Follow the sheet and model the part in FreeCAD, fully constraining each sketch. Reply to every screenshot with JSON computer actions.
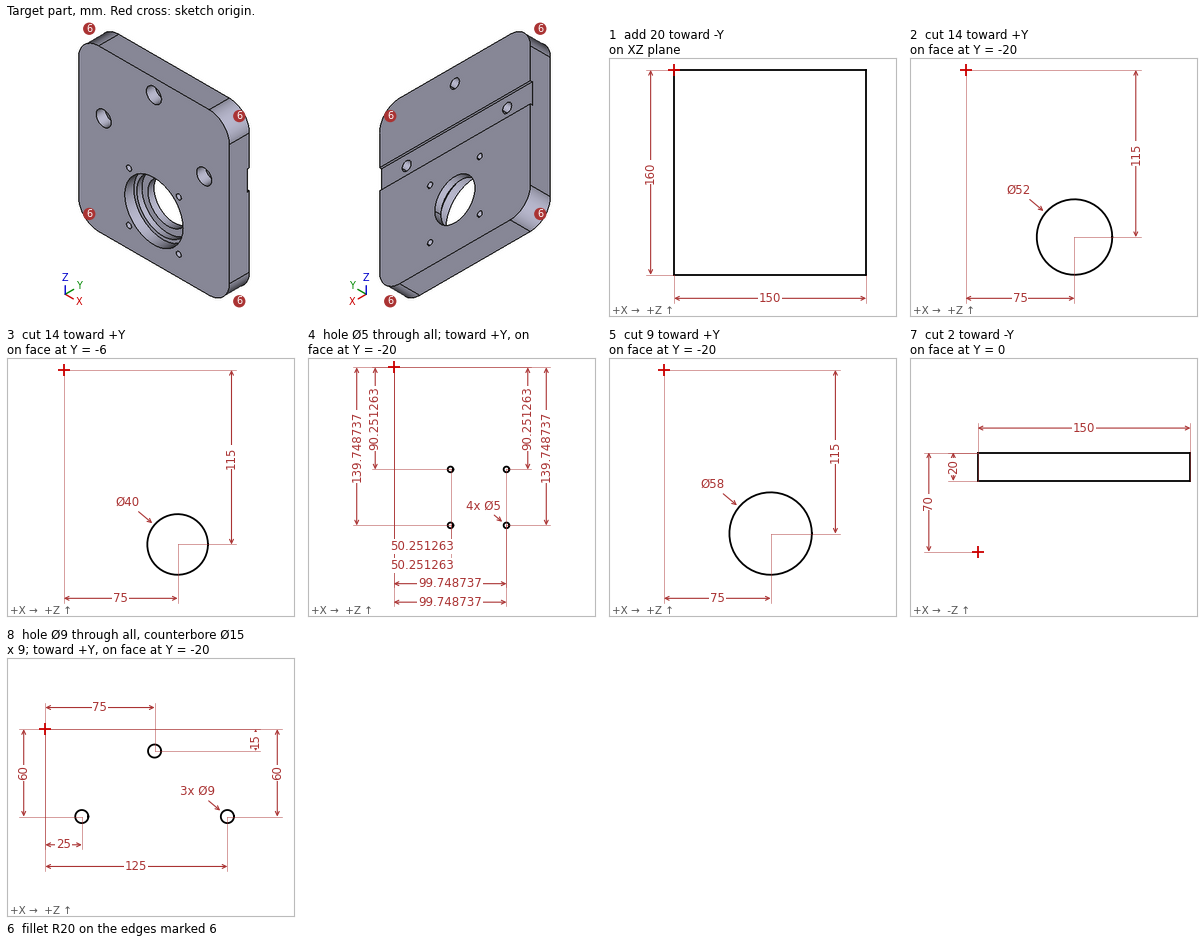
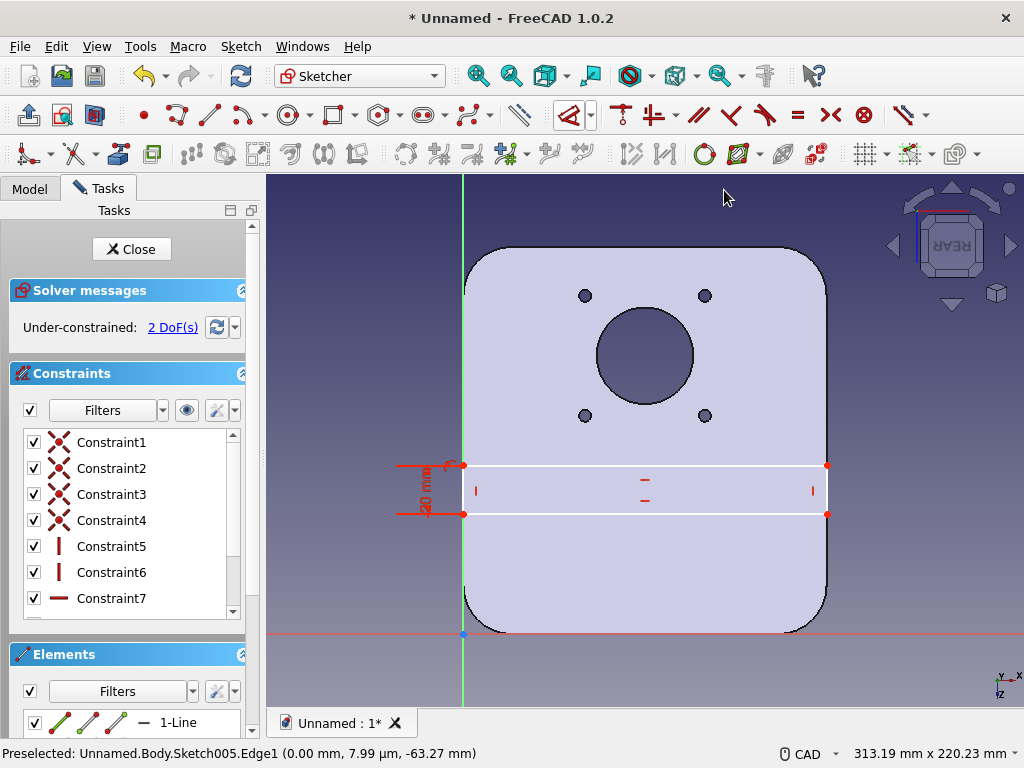
{"action": "left_click", "coordinate": [573, 514]}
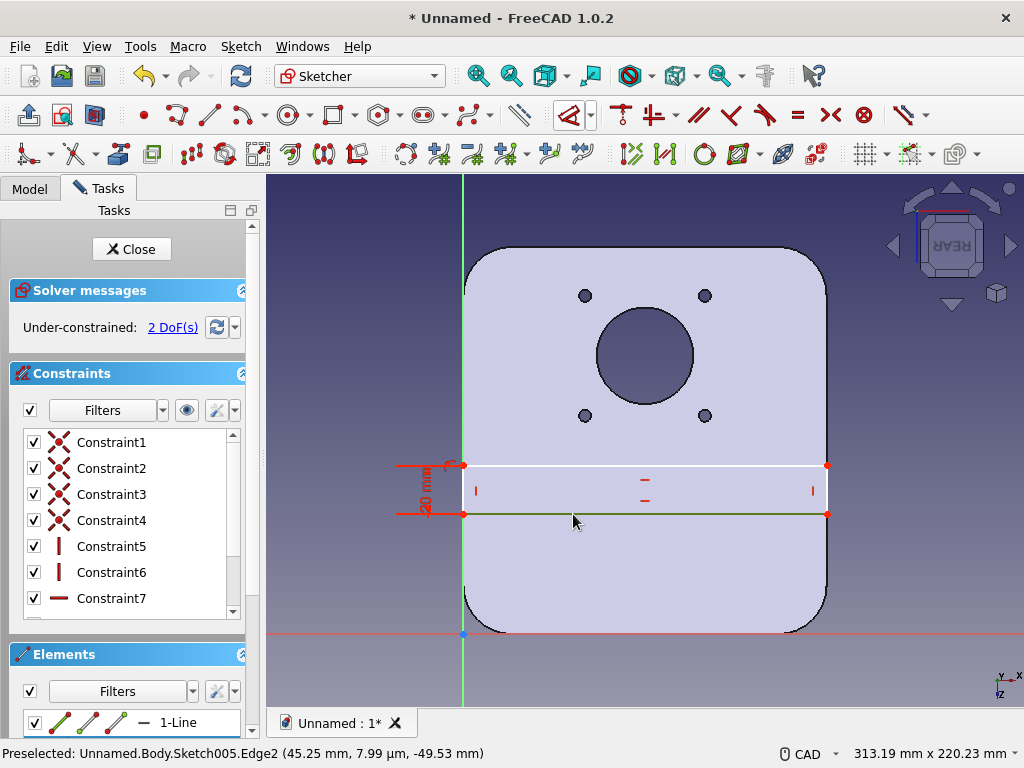
{"action": "left_click", "coordinate": [590, 116]}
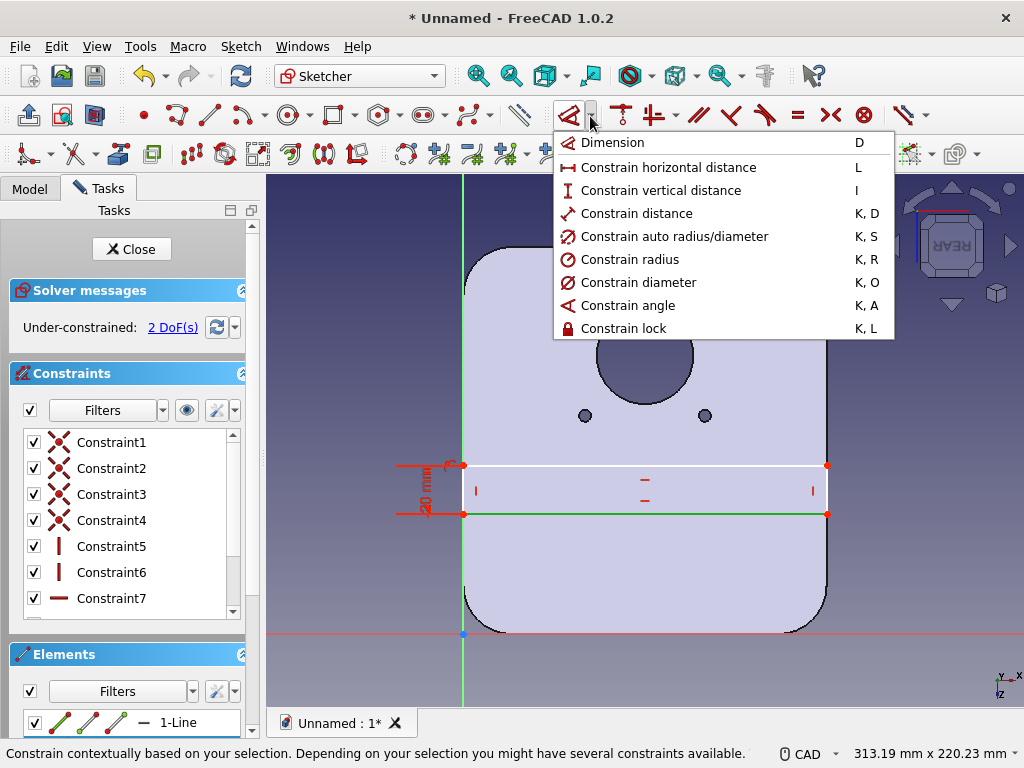
{"action": "left_click", "coordinate": [724, 168]}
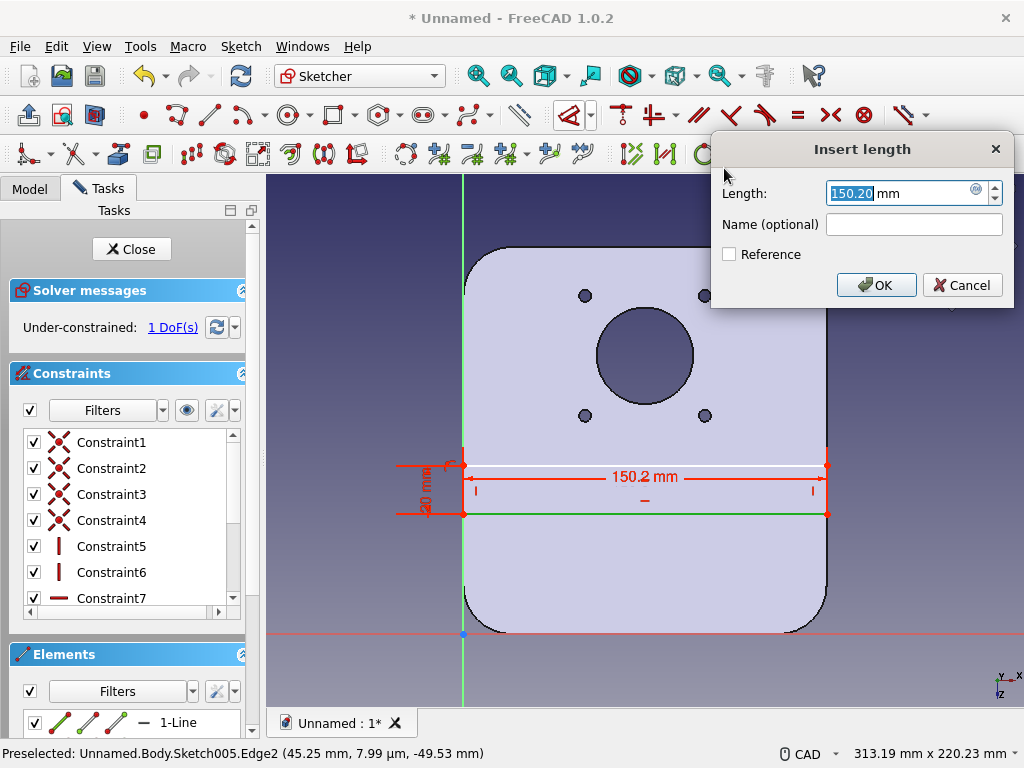
{"action": "type", "text": "150"}
{"action": "key", "text": "Return"}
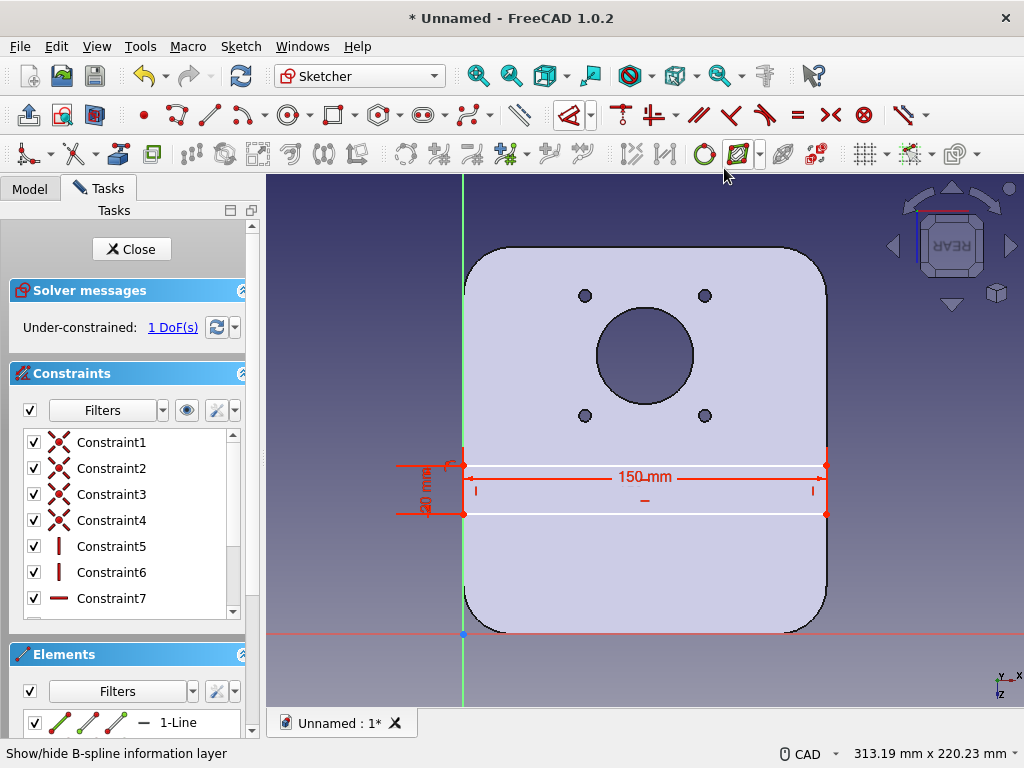
{"action": "left_click", "coordinate": [463, 466]}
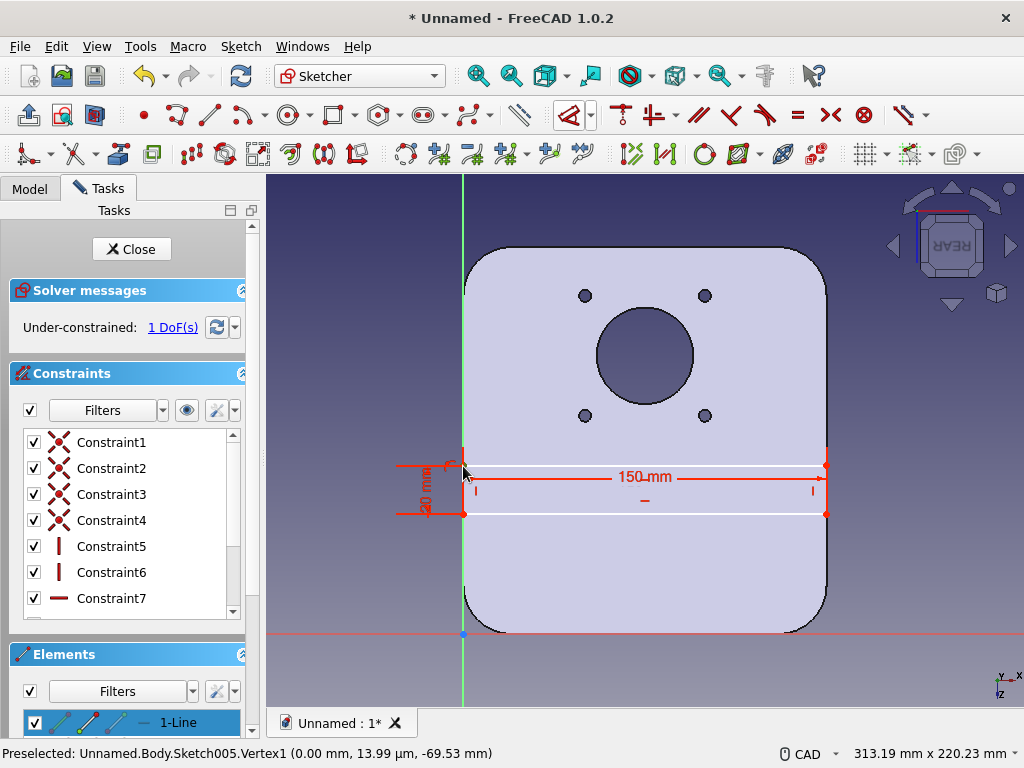
{"action": "key", "text": "i"}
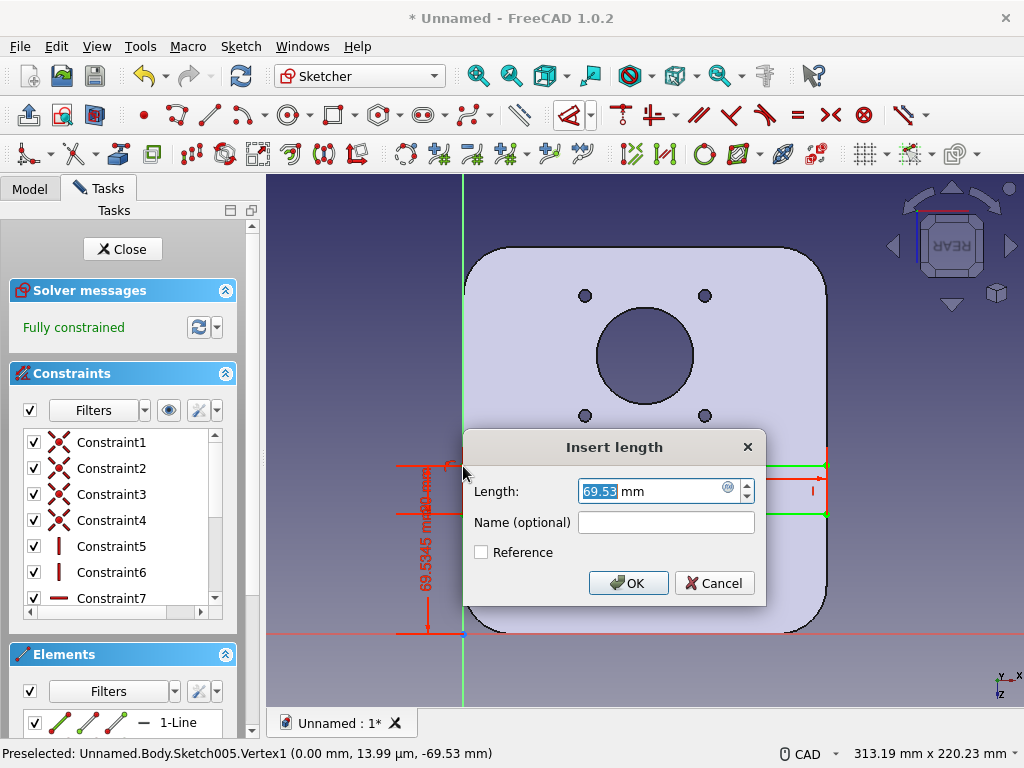
{"action": "type", "text": "70"}
{"action": "key", "text": "Return"}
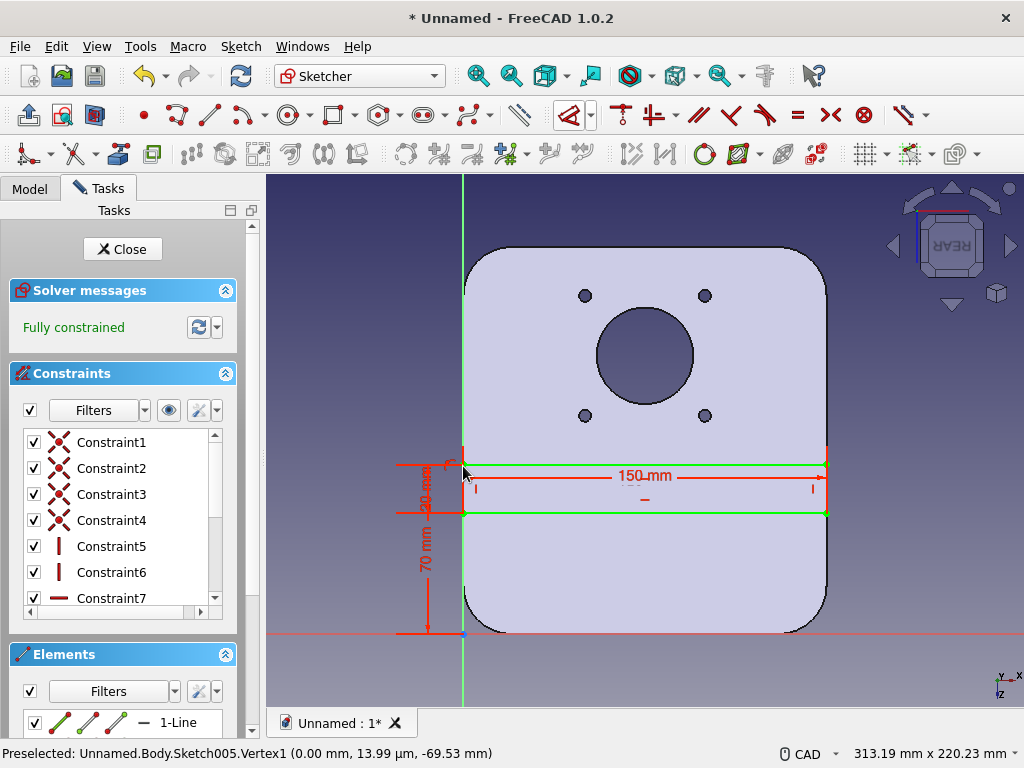
{"action": "left_click", "coordinate": [123, 249]}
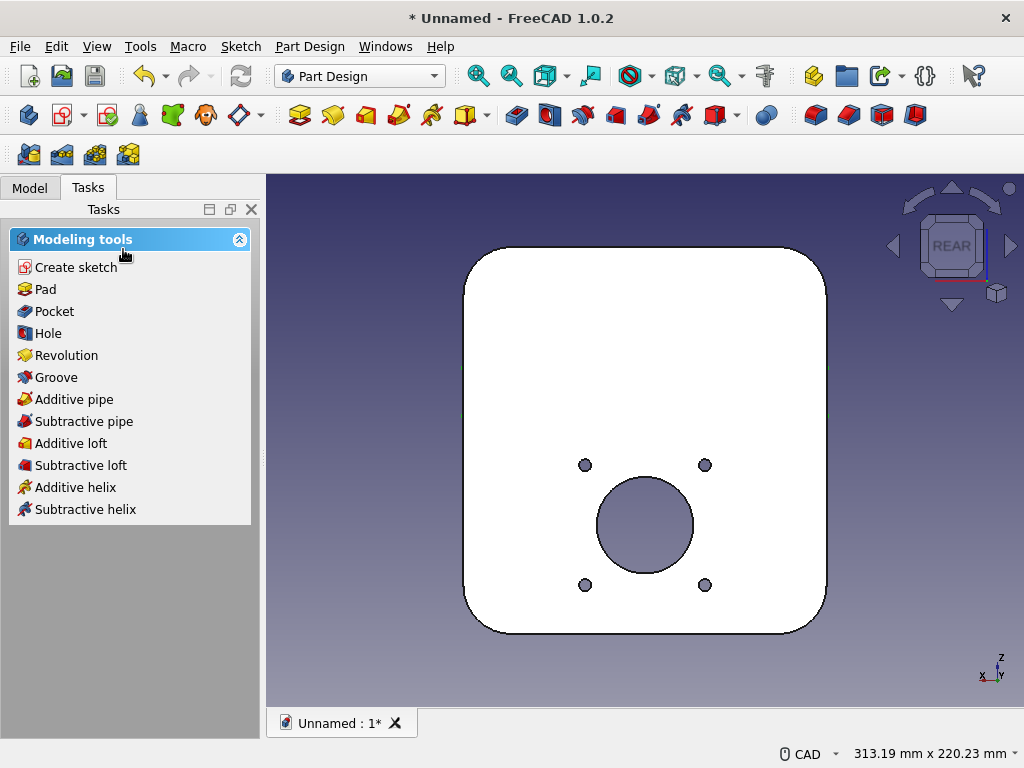
{"action": "left_click", "coordinate": [517, 116]}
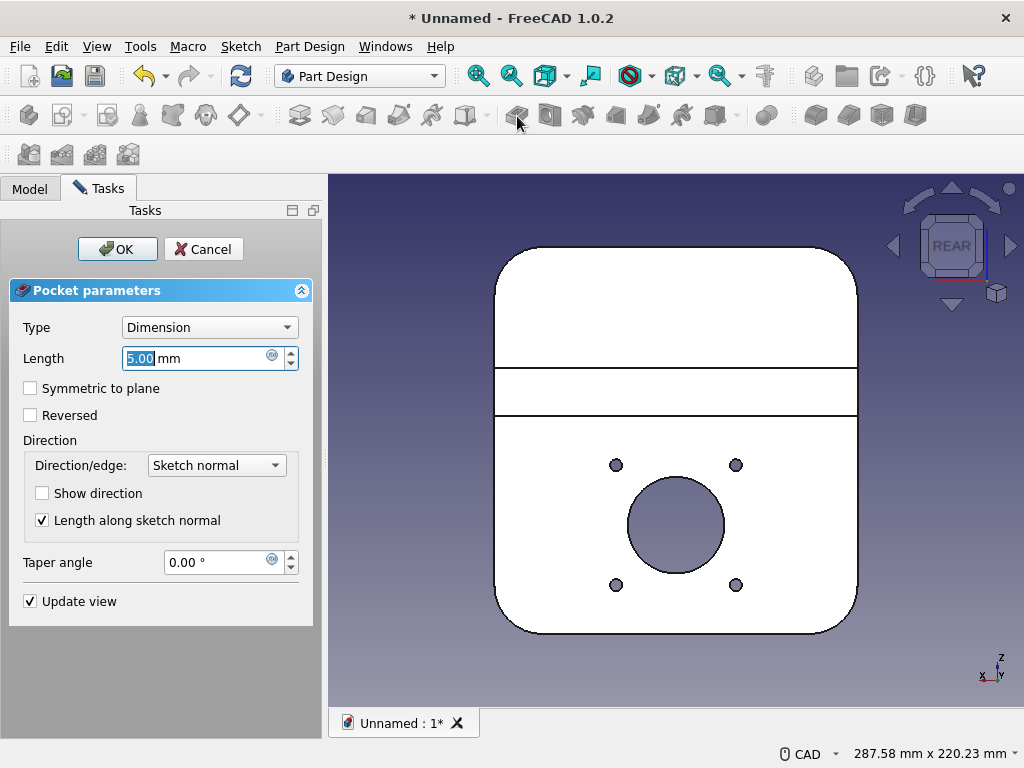
{"action": "type", "text": "2"}
{"action": "key", "text": "Tab"}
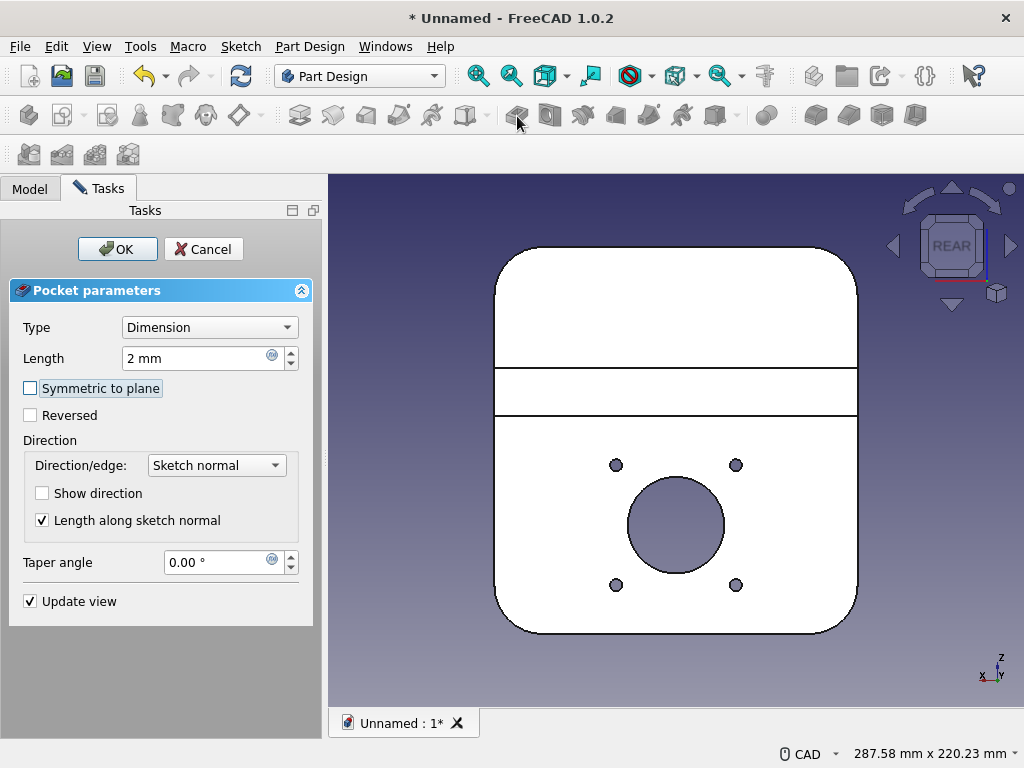
{"action": "left_click", "coordinate": [118, 249]}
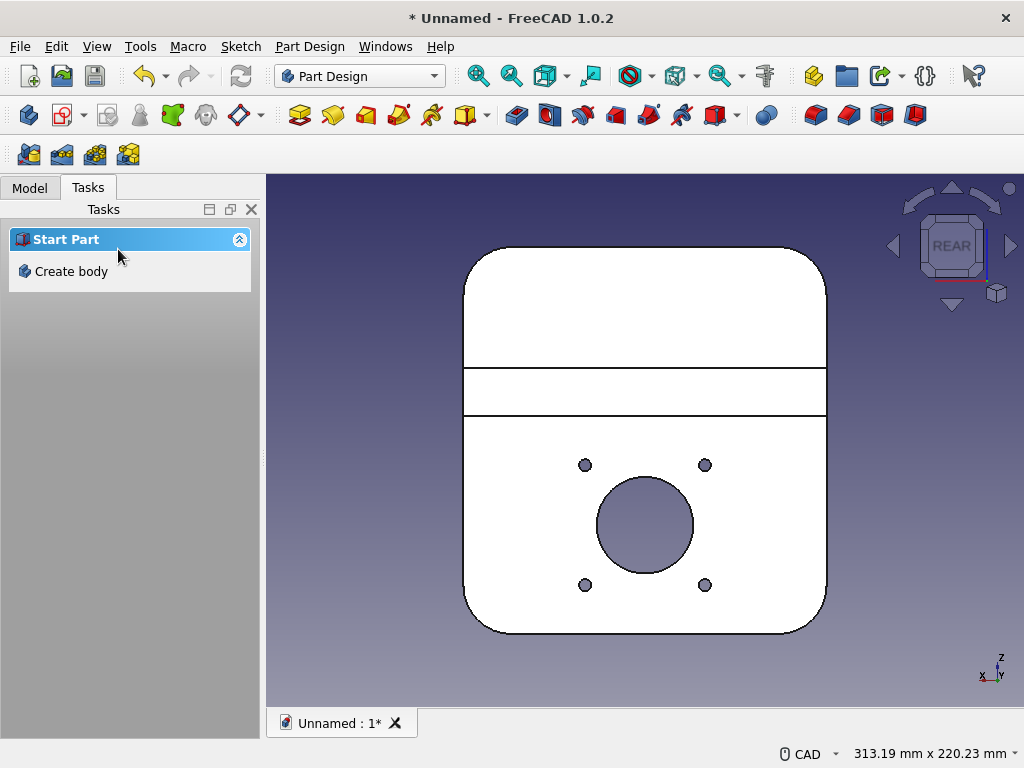
{"action": "key", "text": "0"}